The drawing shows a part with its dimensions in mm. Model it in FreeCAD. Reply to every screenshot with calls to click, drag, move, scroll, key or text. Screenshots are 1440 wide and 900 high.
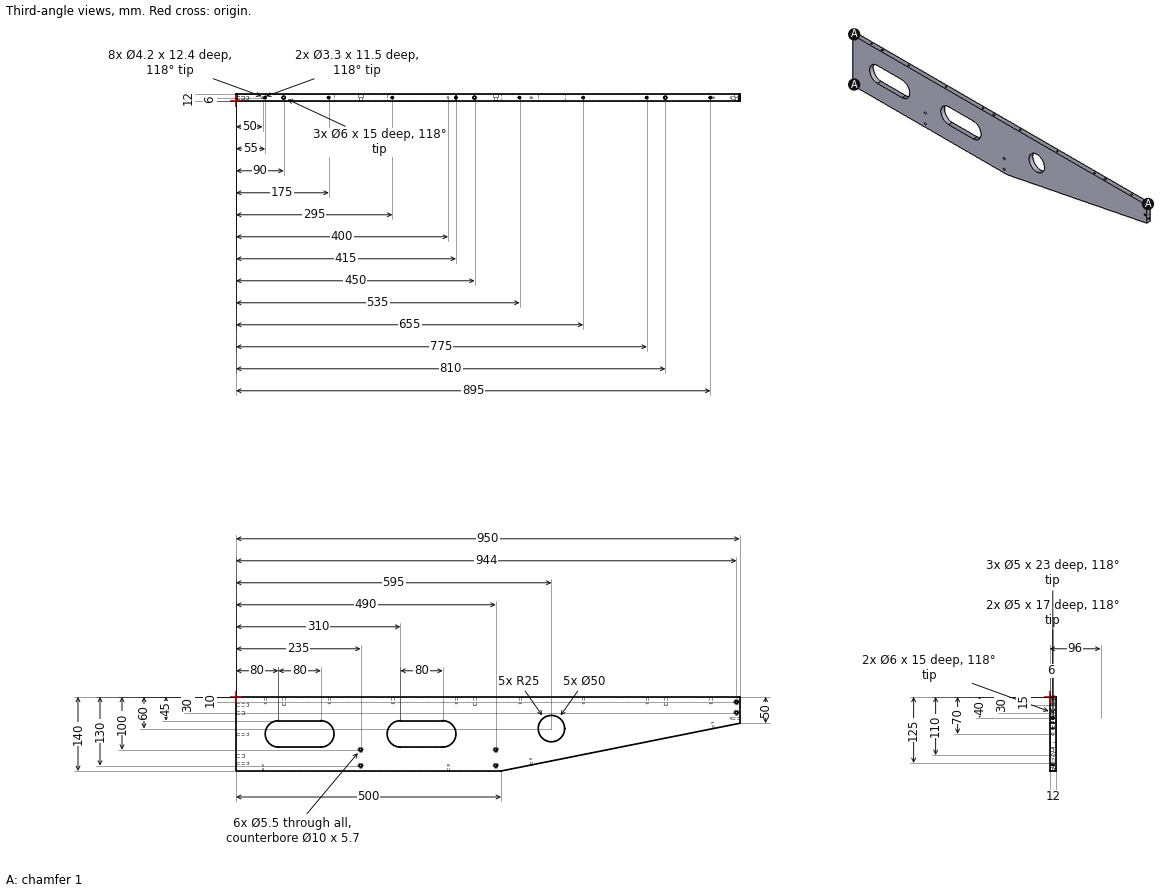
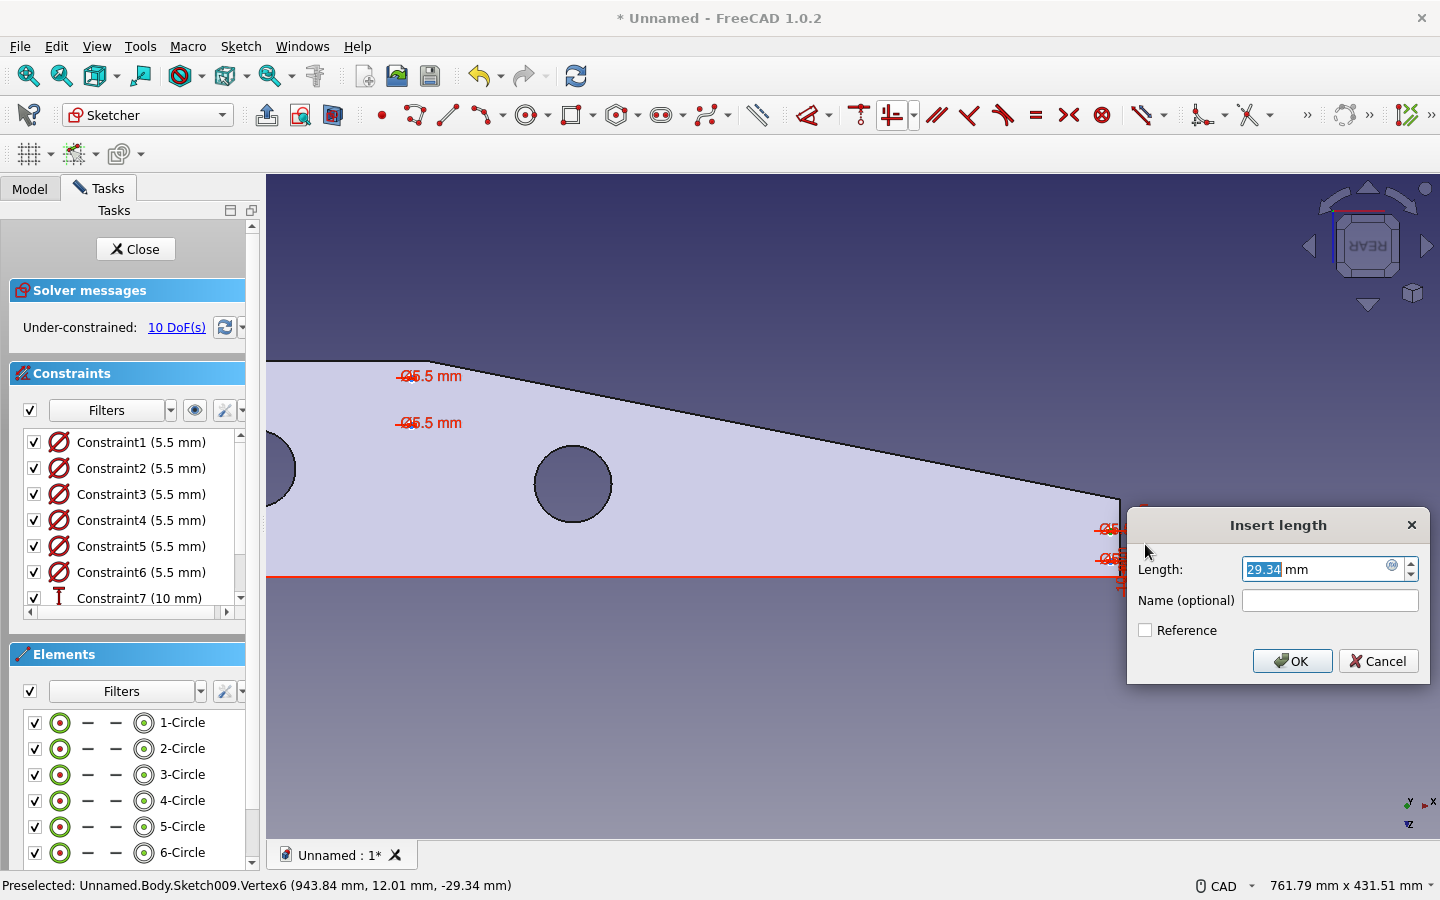
text(30)
key(Return)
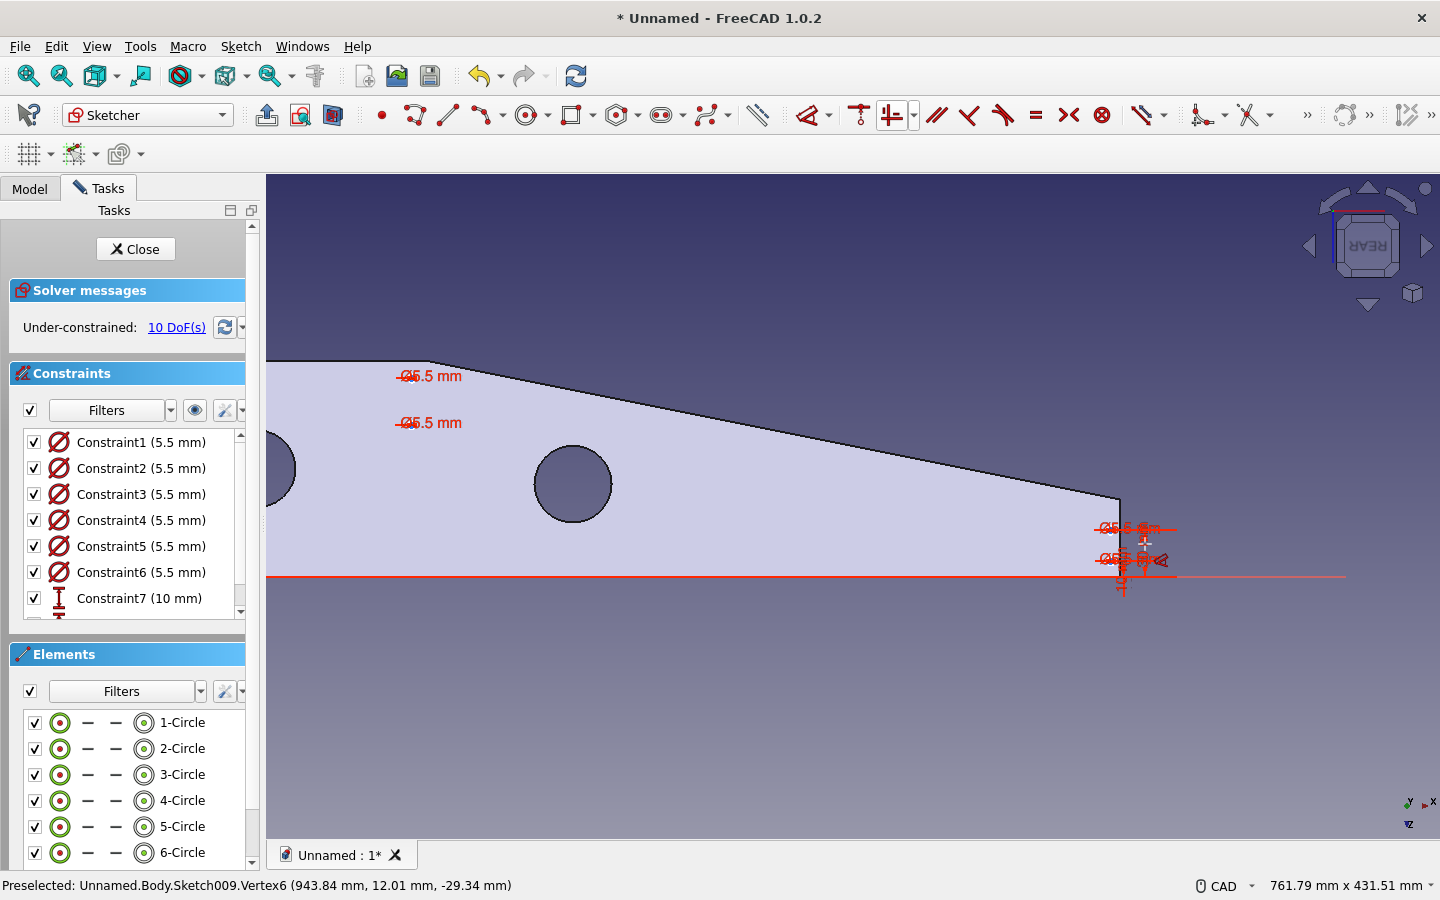
scroll(1110, 533, down, 4)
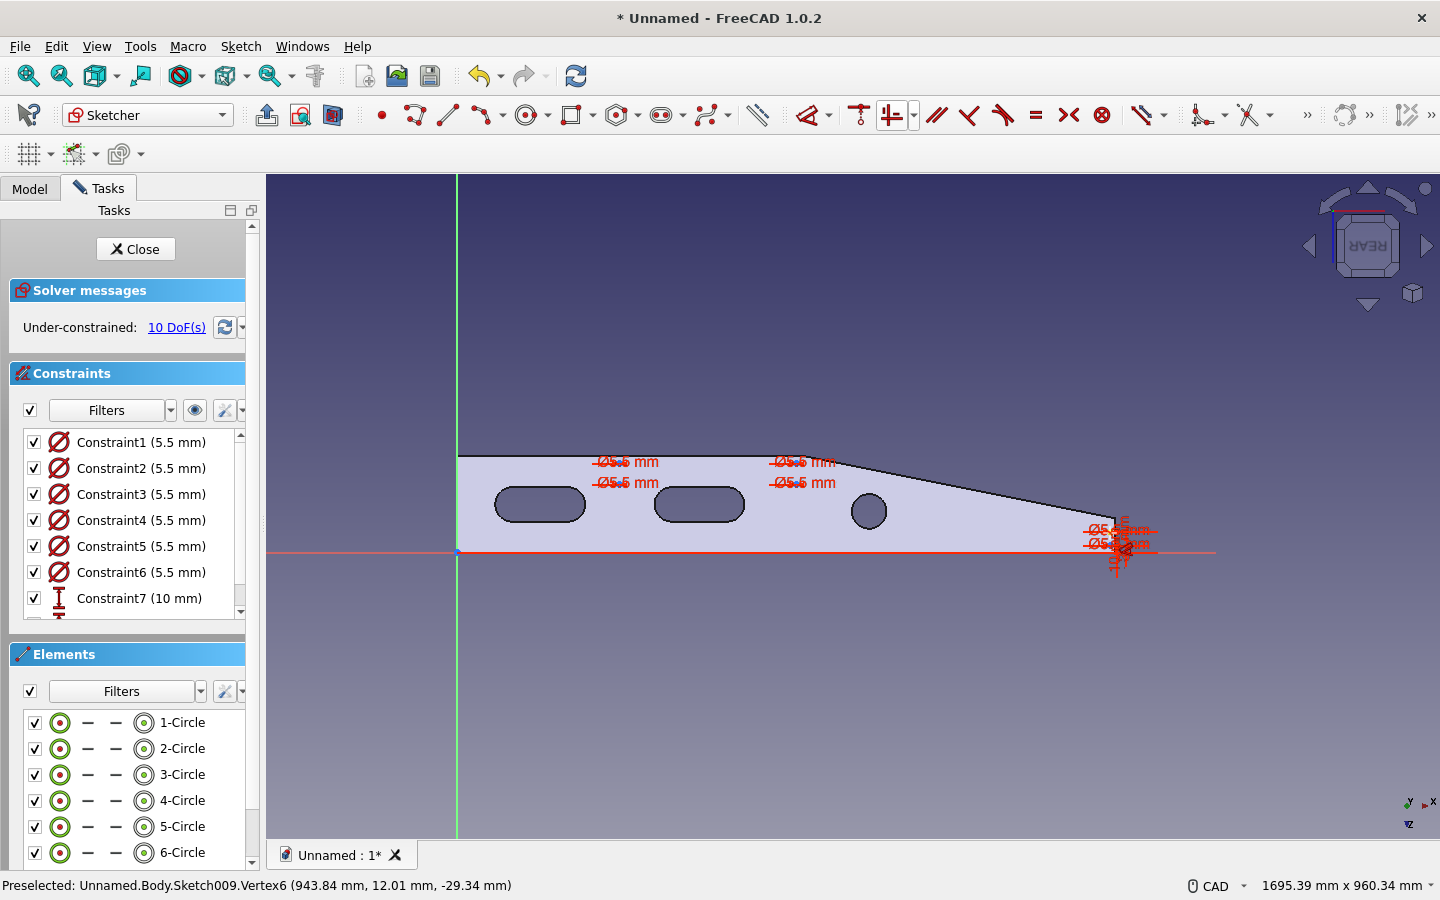
click(620, 485)
click(538, 587)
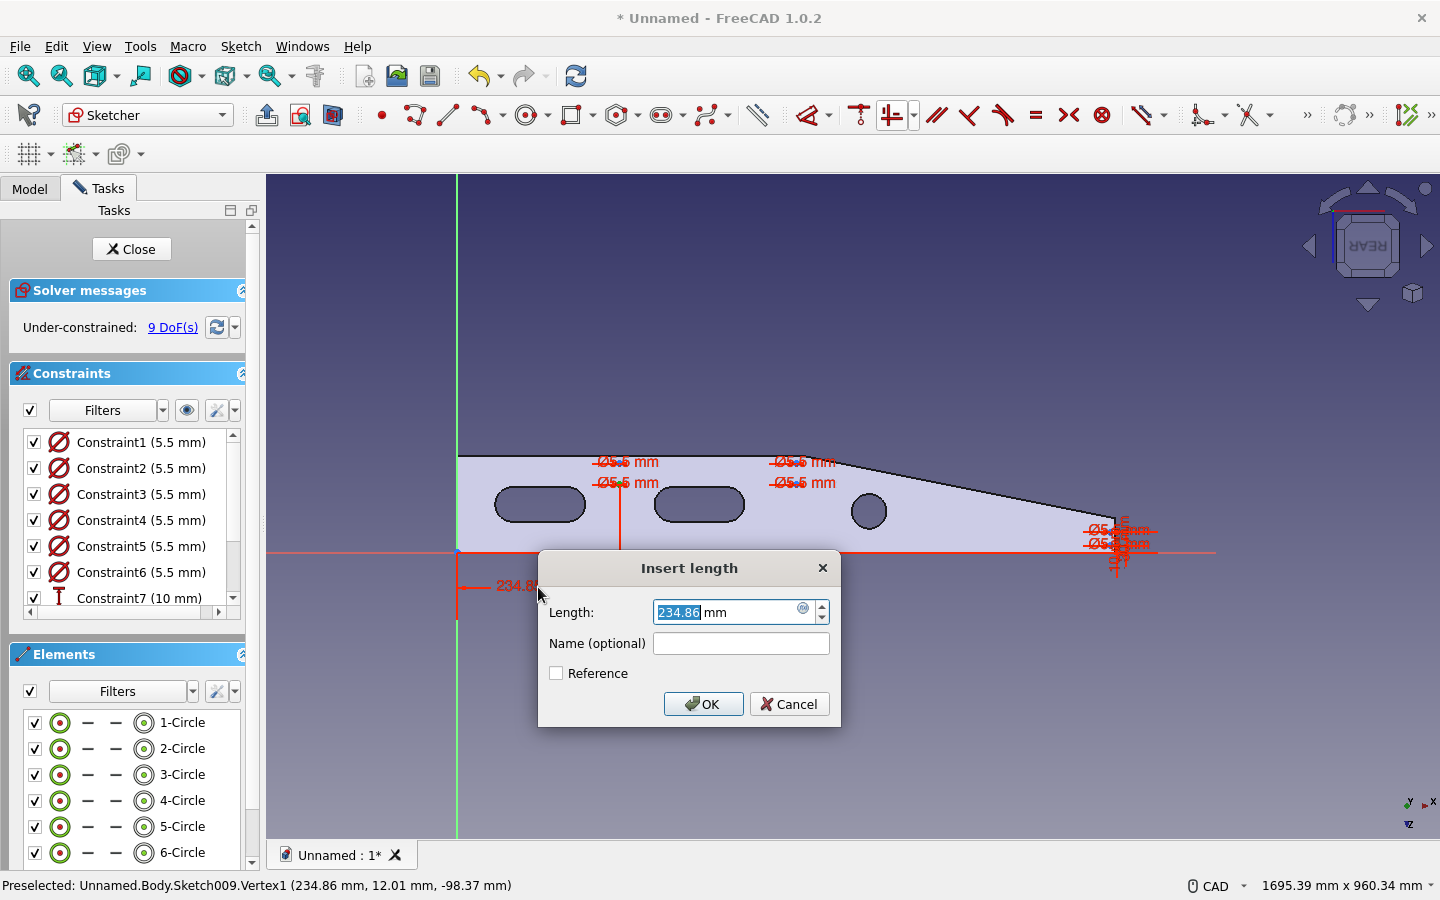
text(235)
key(Return)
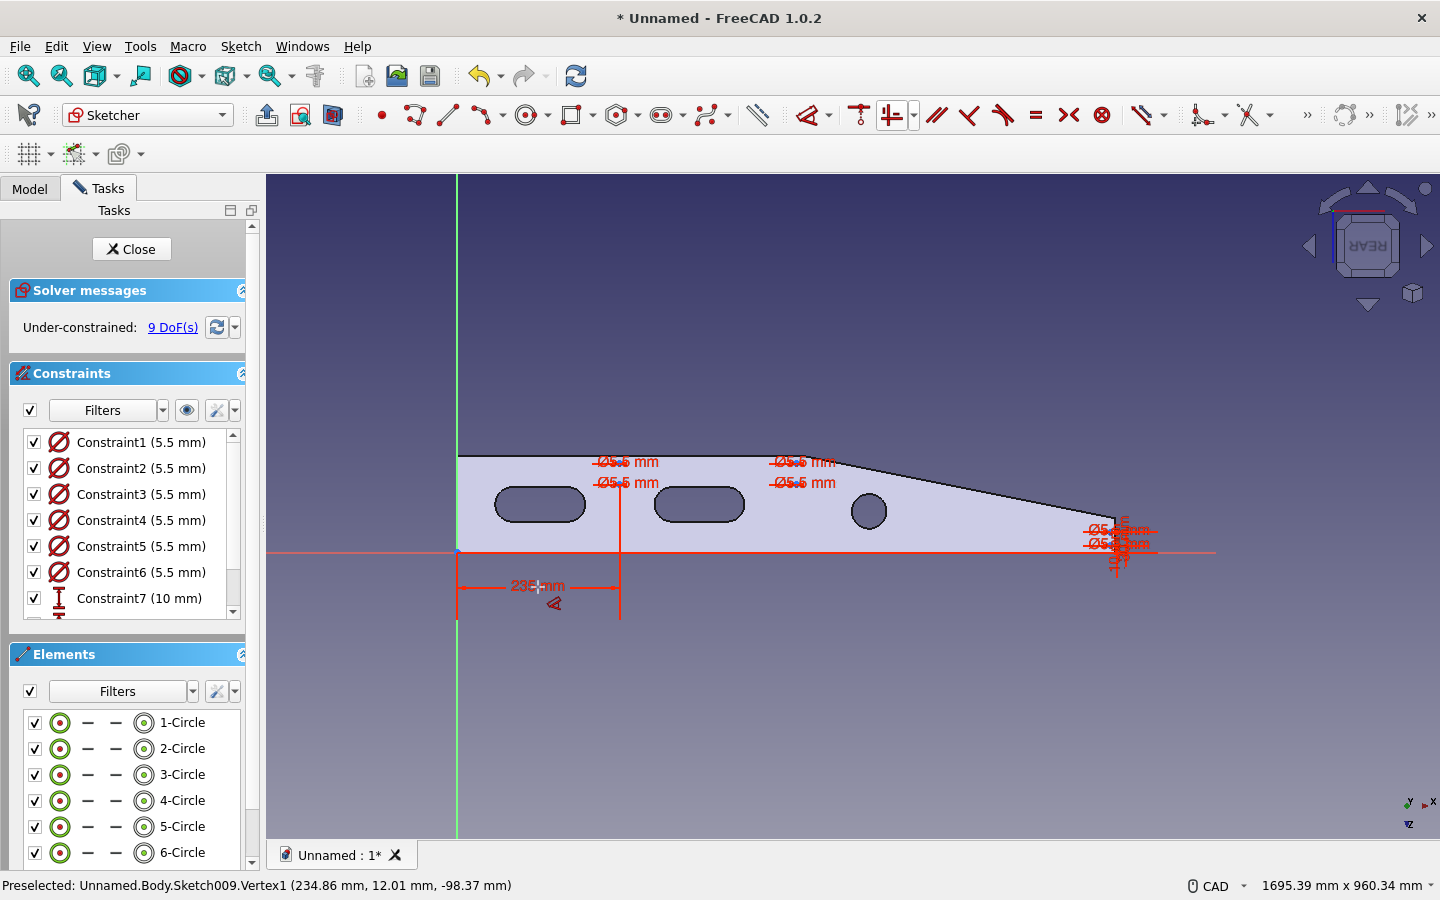
click(620, 485)
click(423, 519)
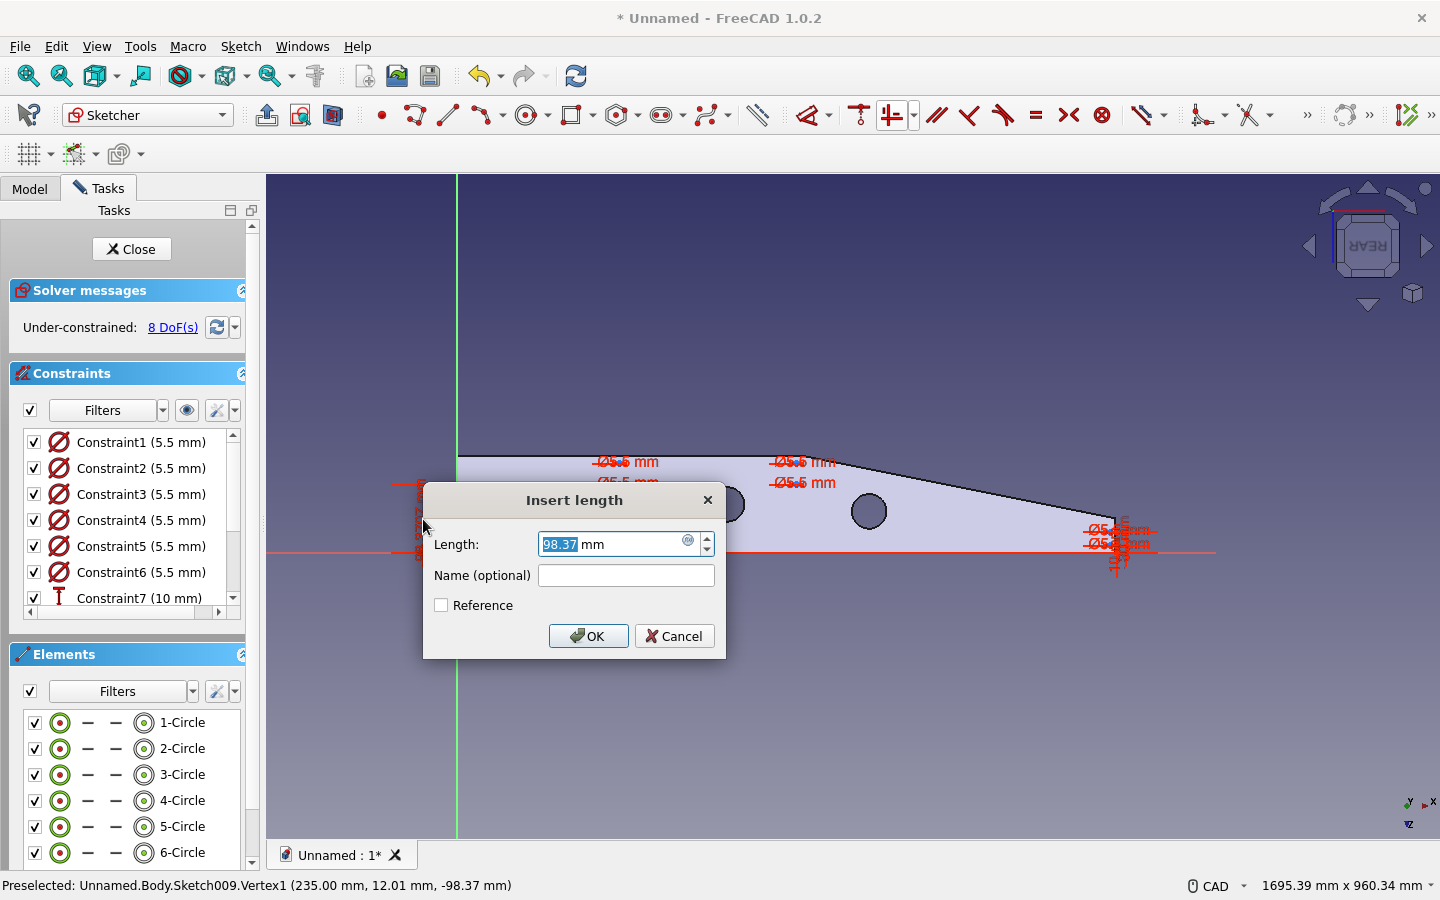
text(100)
key(Return)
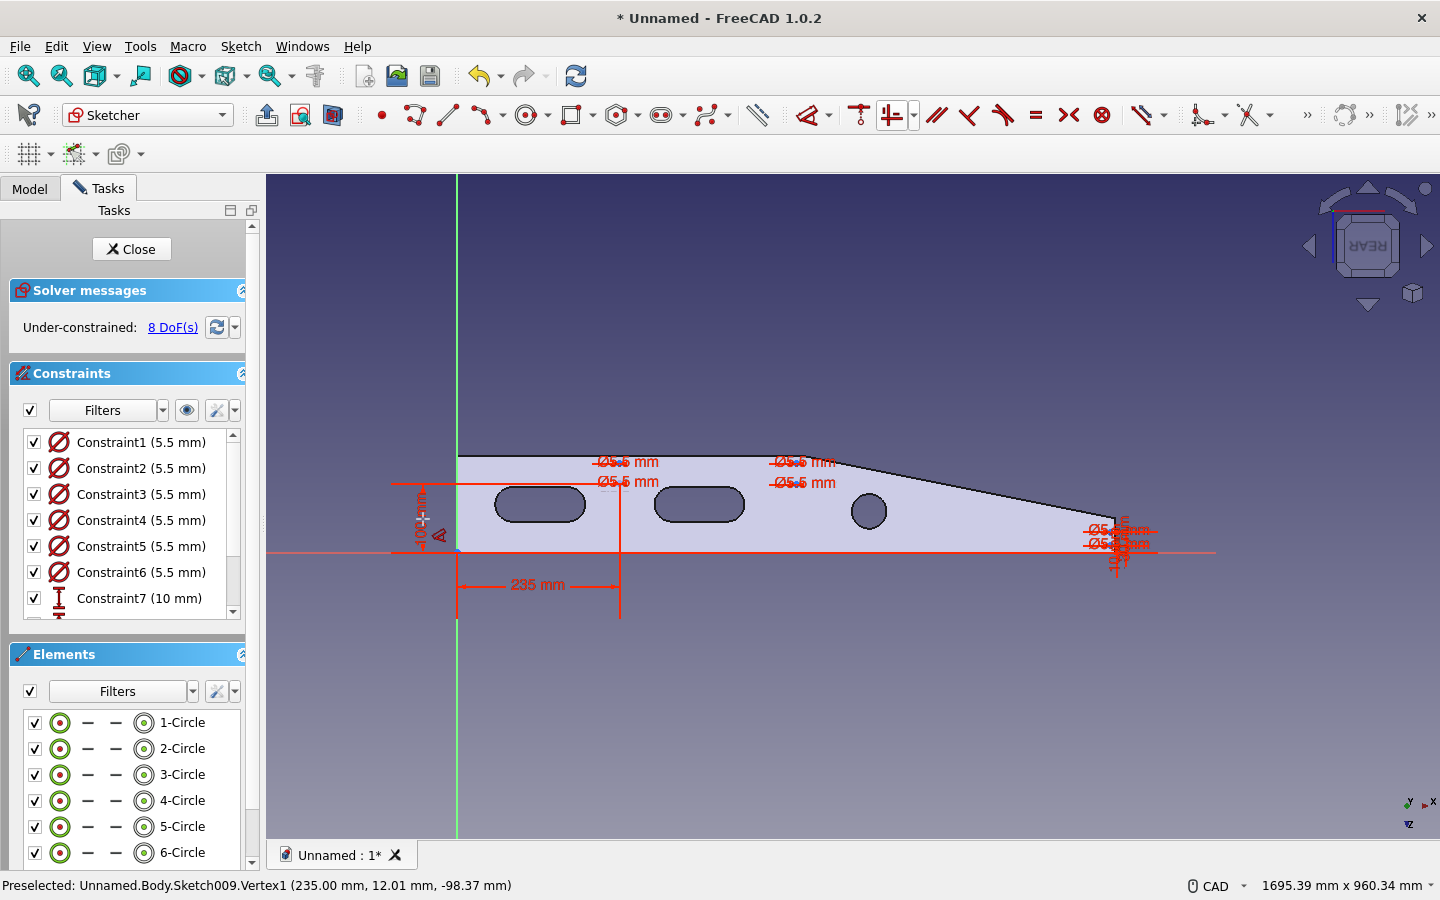
click(620, 464)
click(538, 430)